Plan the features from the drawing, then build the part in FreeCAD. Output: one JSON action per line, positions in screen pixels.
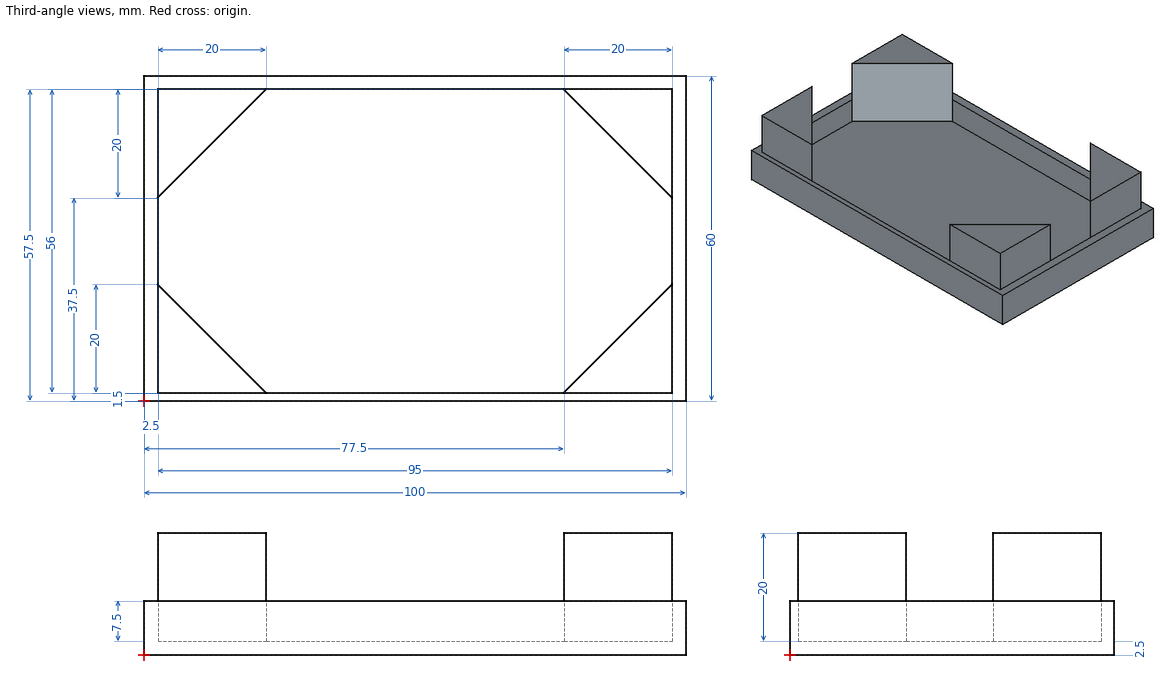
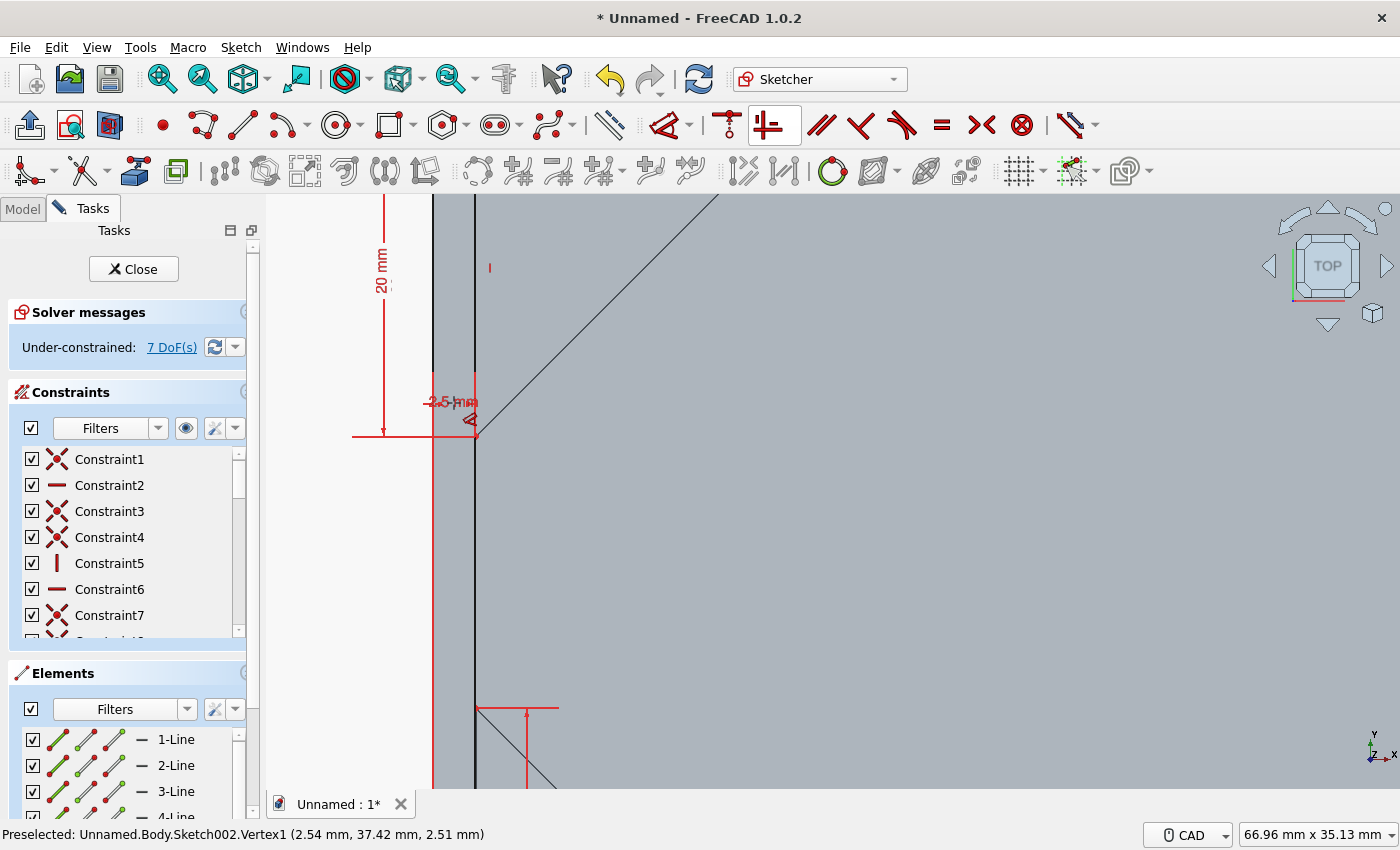
{"action": "scroll", "coordinate": [477, 438], "scroll_direction": "down", "scroll_amount": 5}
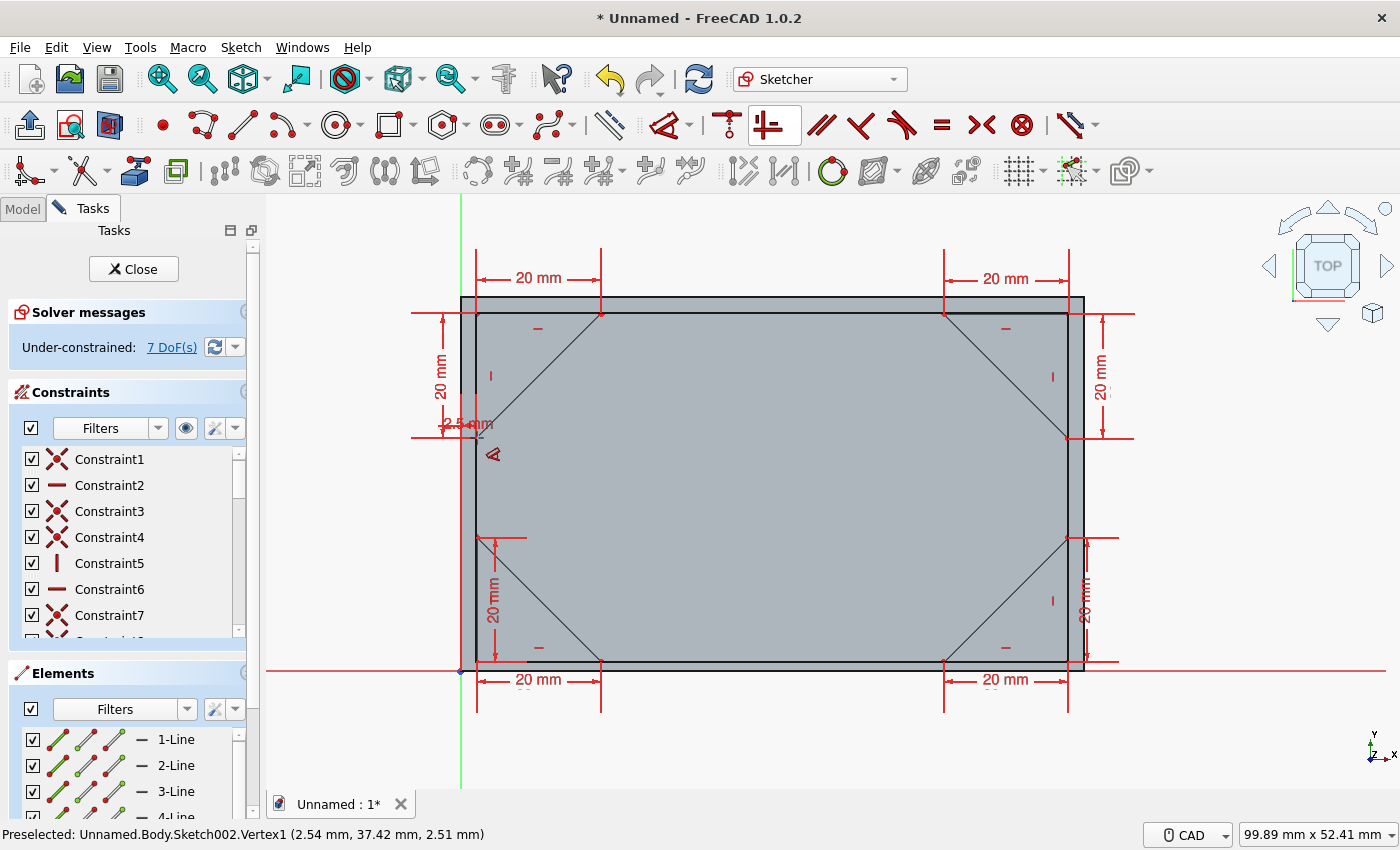
{"action": "scroll", "coordinate": [477, 662], "scroll_direction": "up", "scroll_amount": 5}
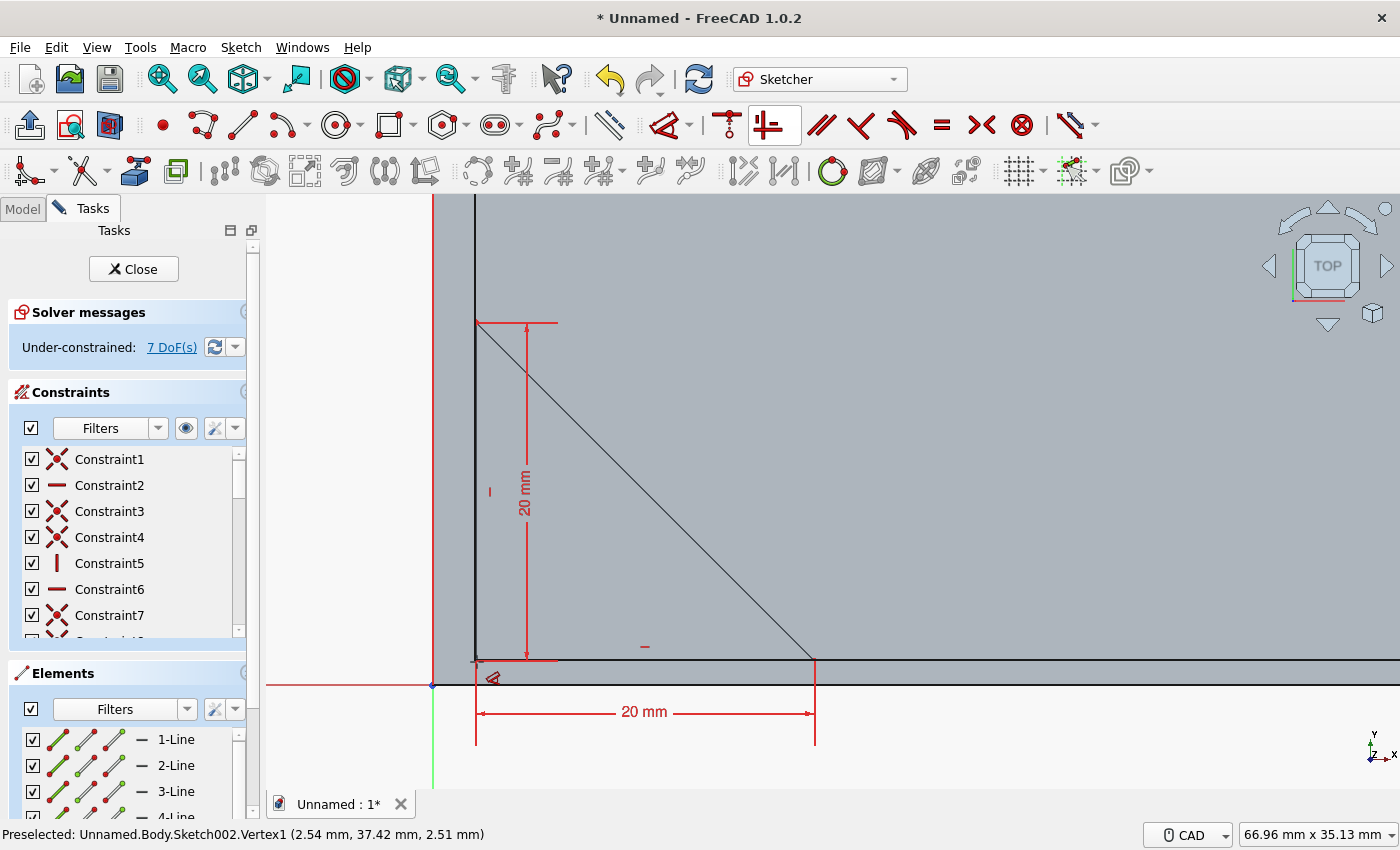
{"action": "left_click", "coordinate": [476, 661]}
{"action": "left_click", "coordinate": [454, 719]}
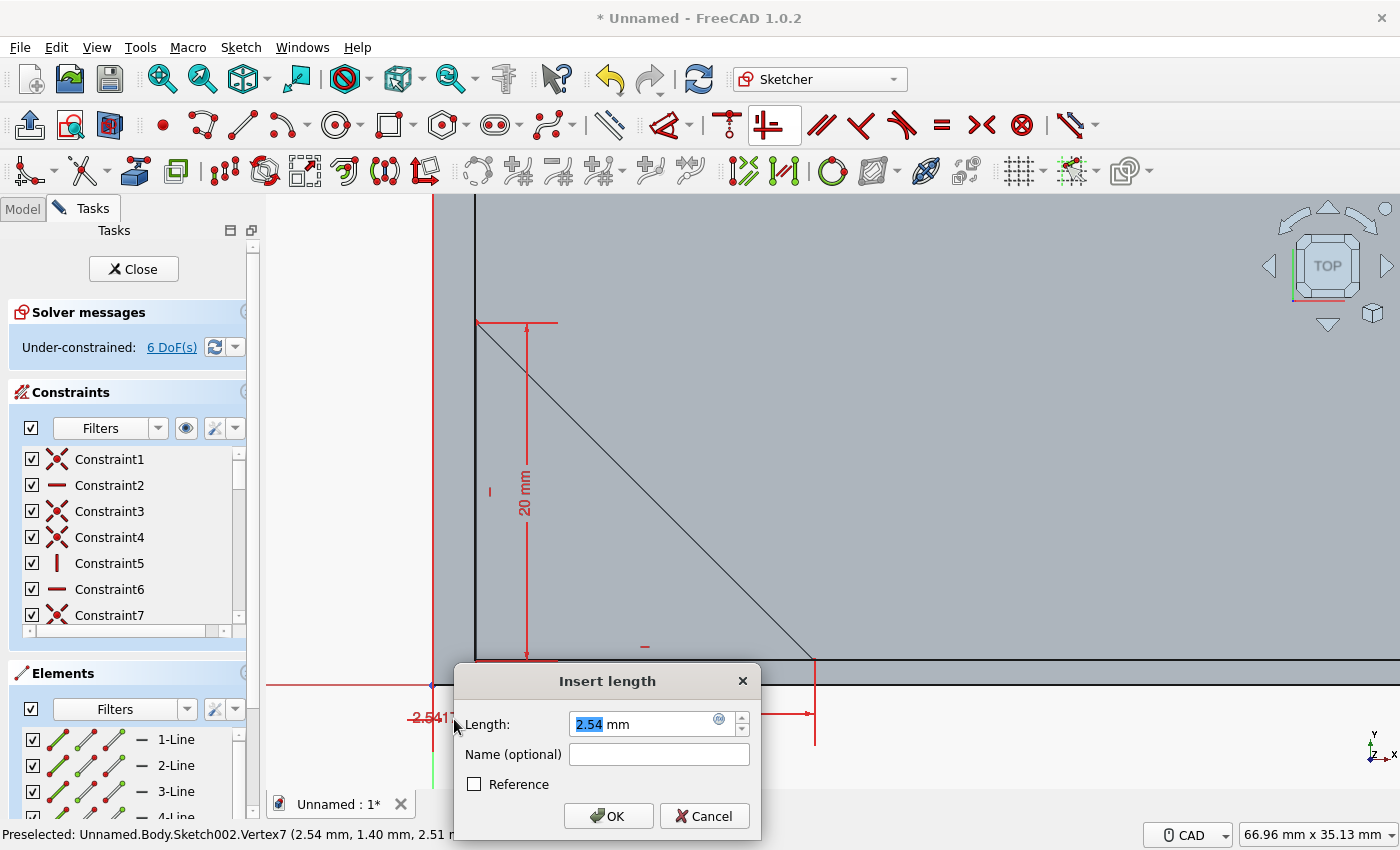
{"action": "type", "text": "2.5"}
{"action": "key", "text": "Return"}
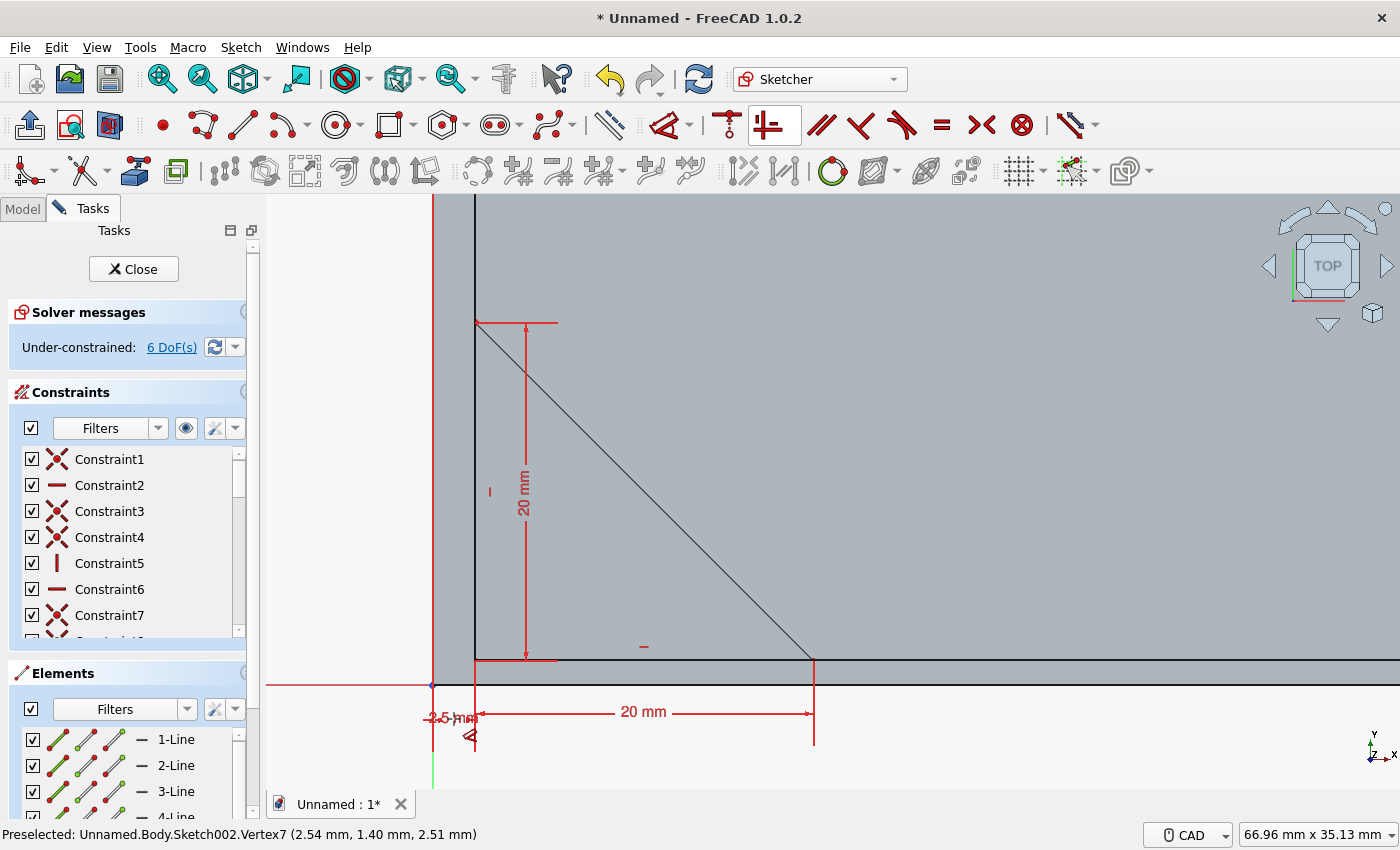
{"action": "scroll", "coordinate": [475, 661], "scroll_direction": "up", "scroll_amount": 3}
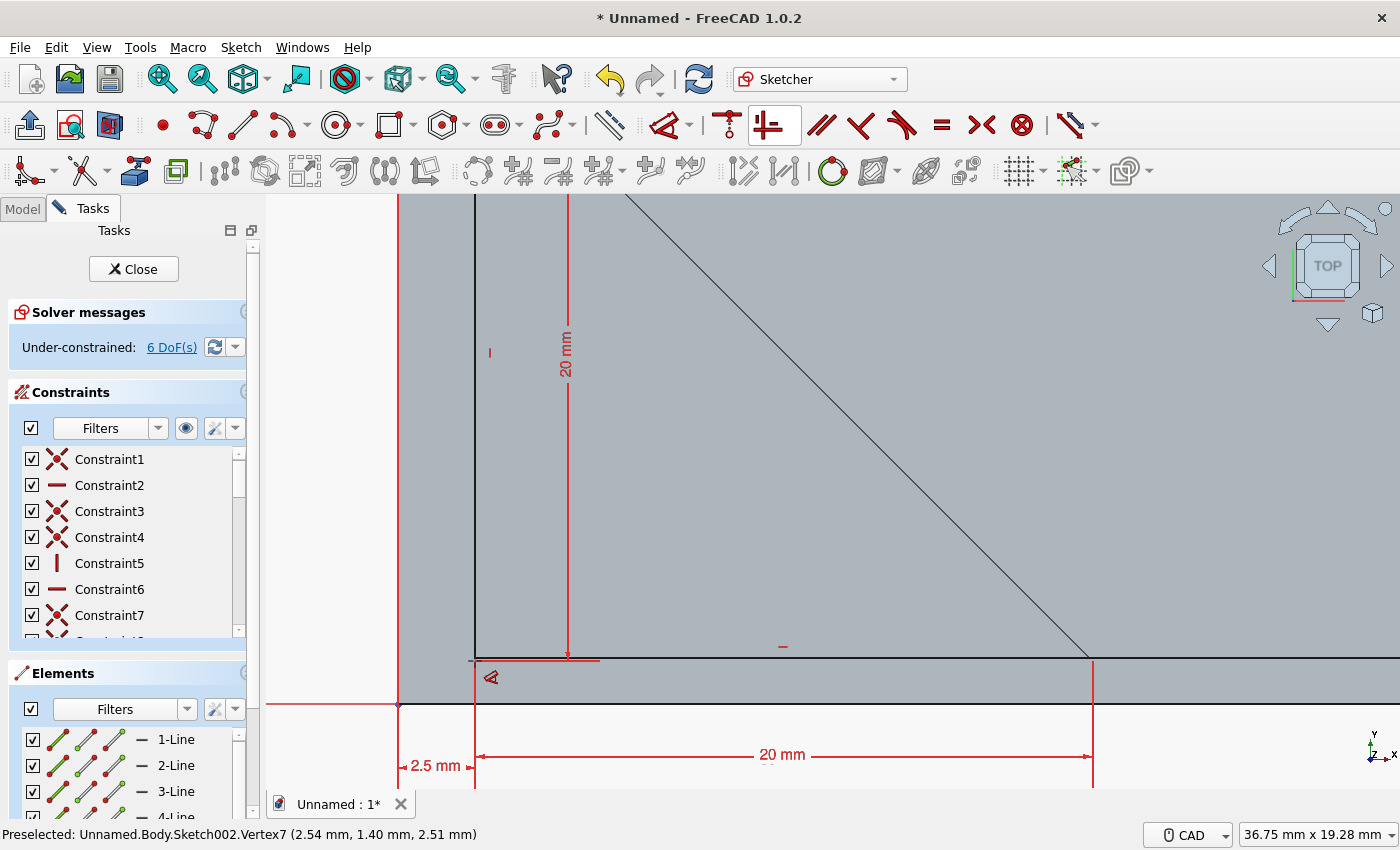
{"action": "left_click", "coordinate": [475, 661]}
{"action": "left_click", "coordinate": [364, 683]}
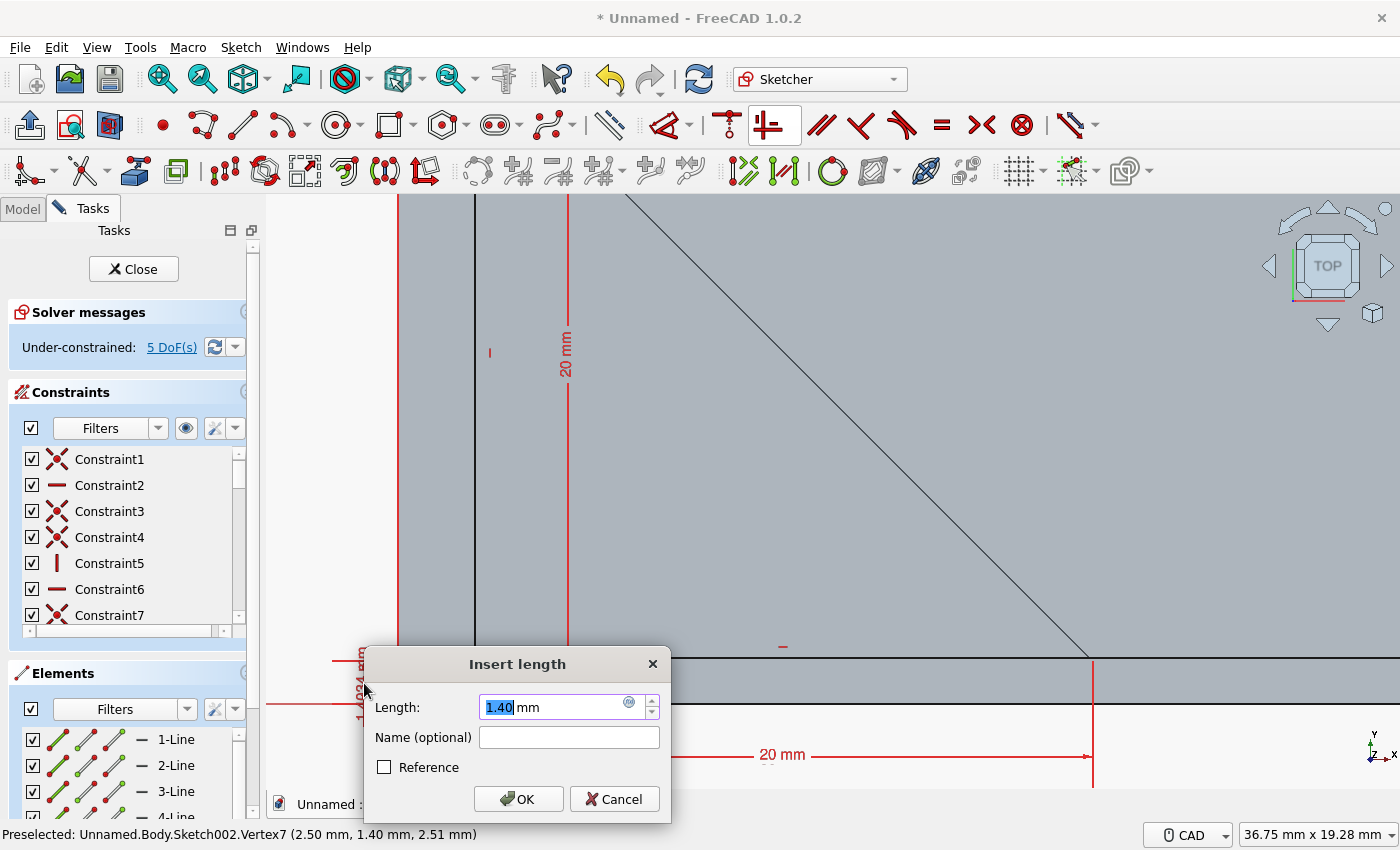
{"action": "type", "text": "1.5"}
{"action": "key", "text": "Return"}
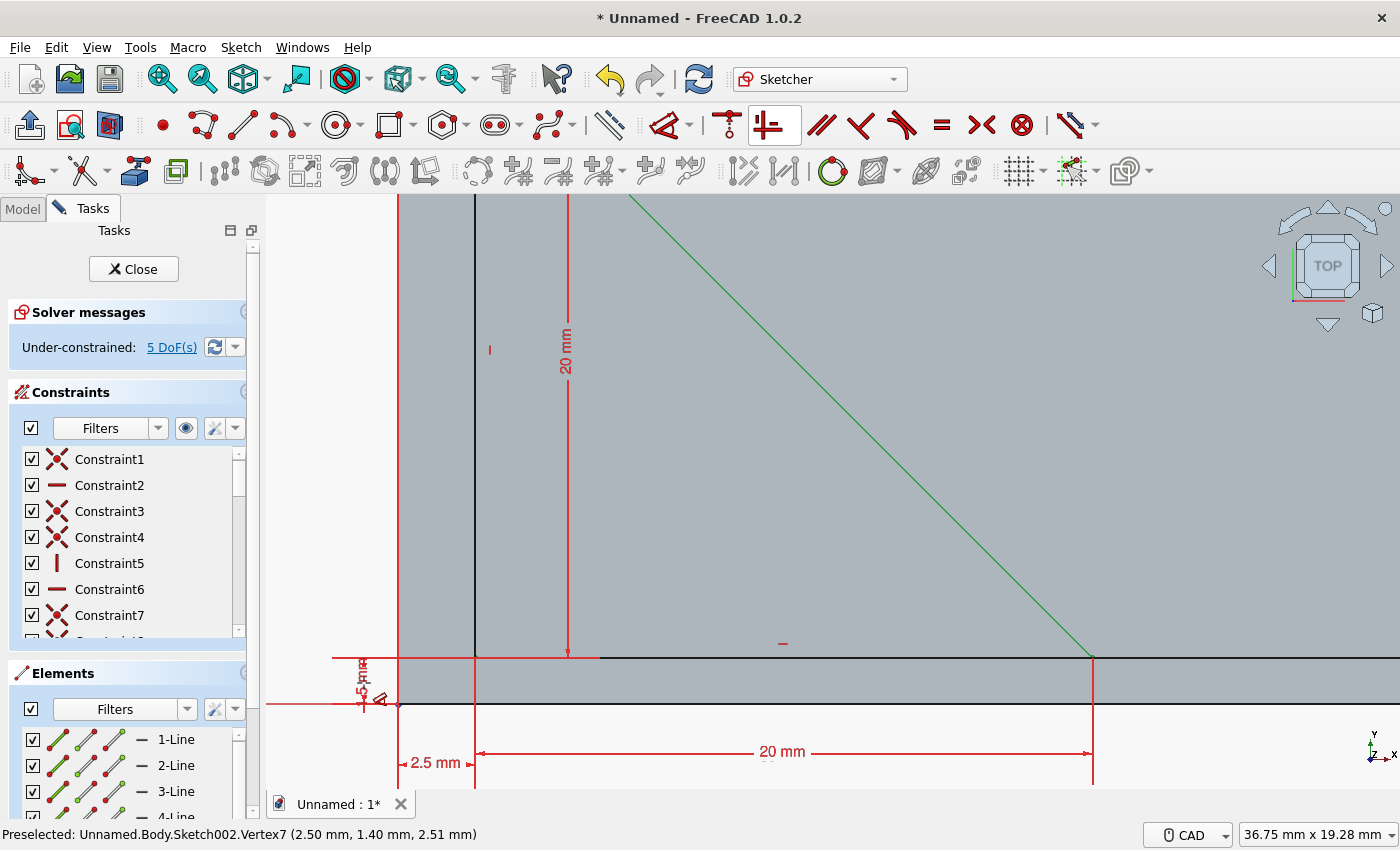
{"action": "scroll", "coordinate": [477, 662], "scroll_direction": "down", "scroll_amount": 8}